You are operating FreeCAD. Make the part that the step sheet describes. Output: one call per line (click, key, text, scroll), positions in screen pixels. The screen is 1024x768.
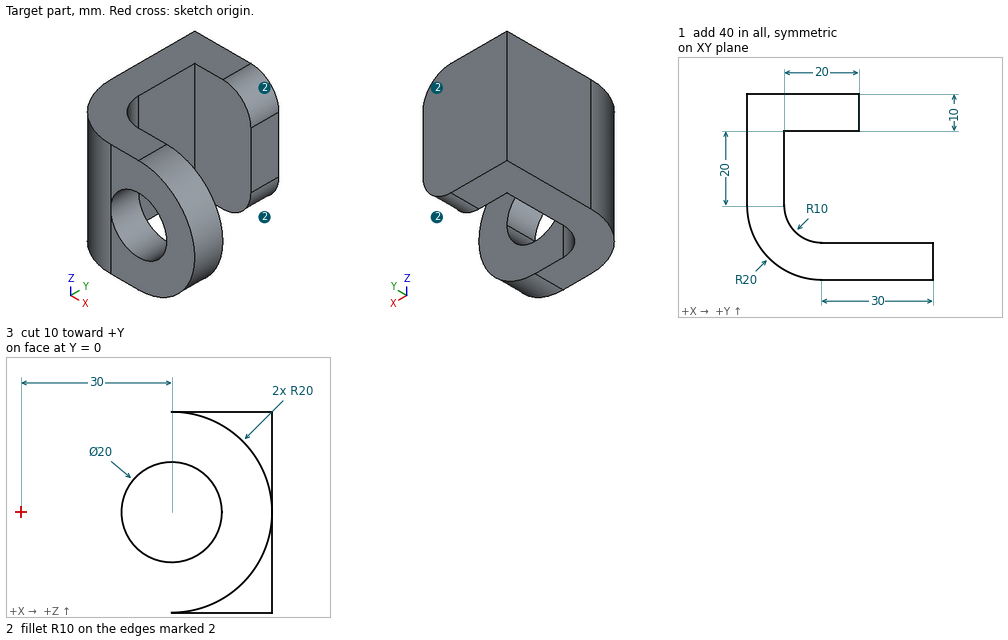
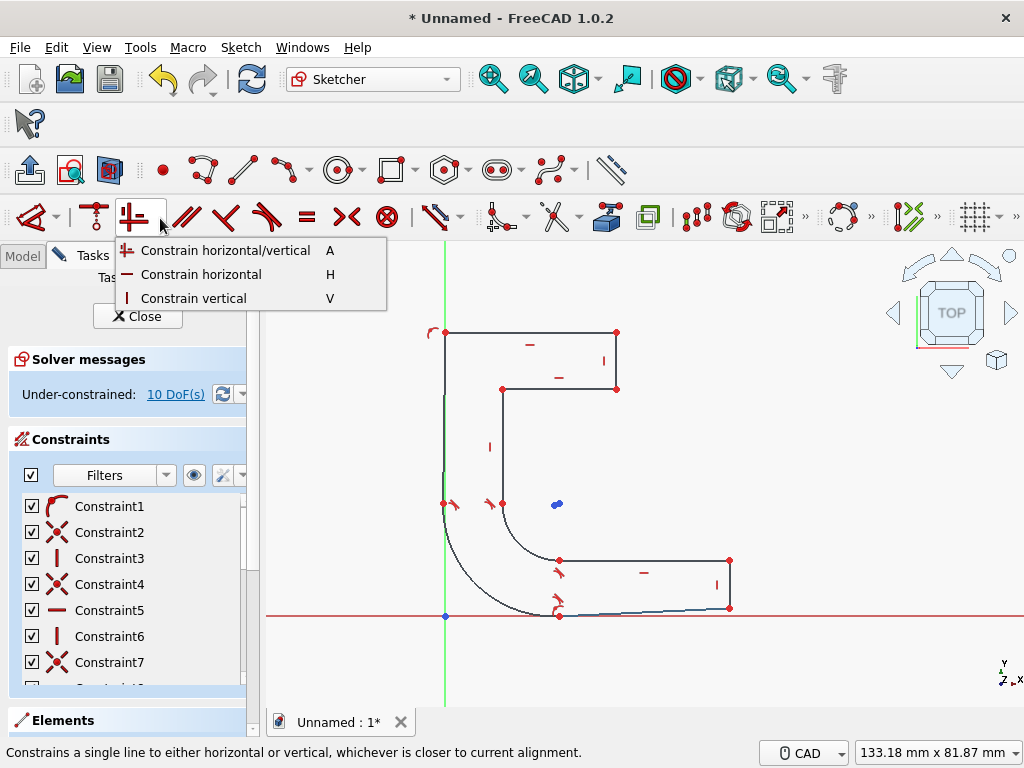
click(251, 274)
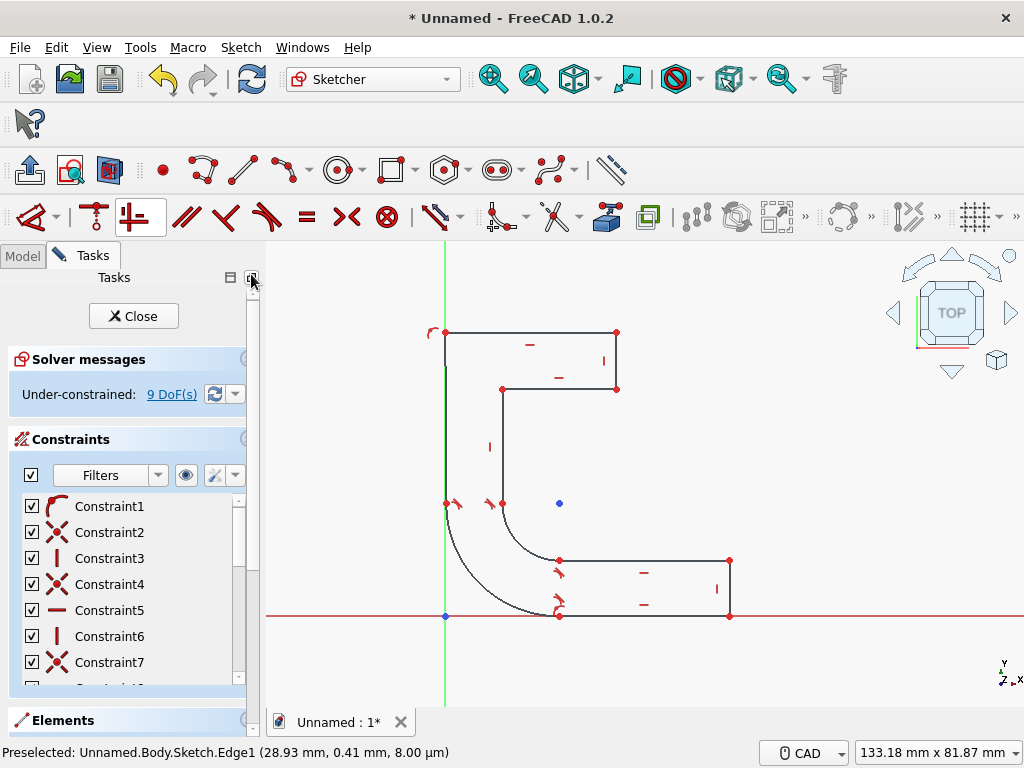
click(446, 384)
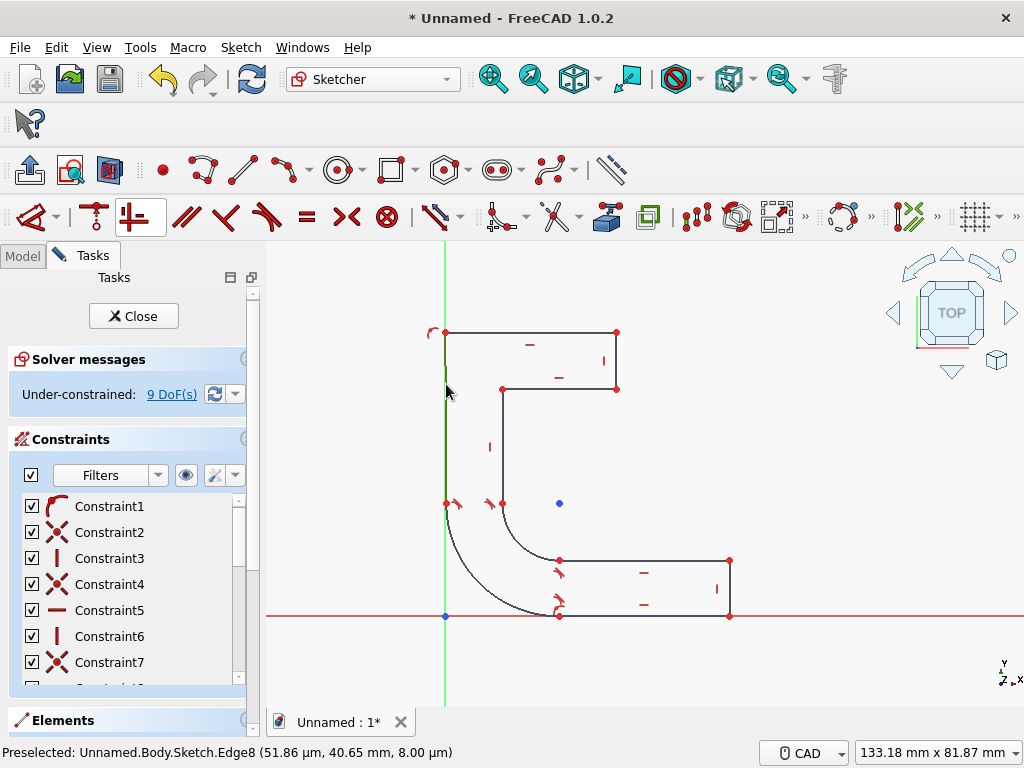
key(v)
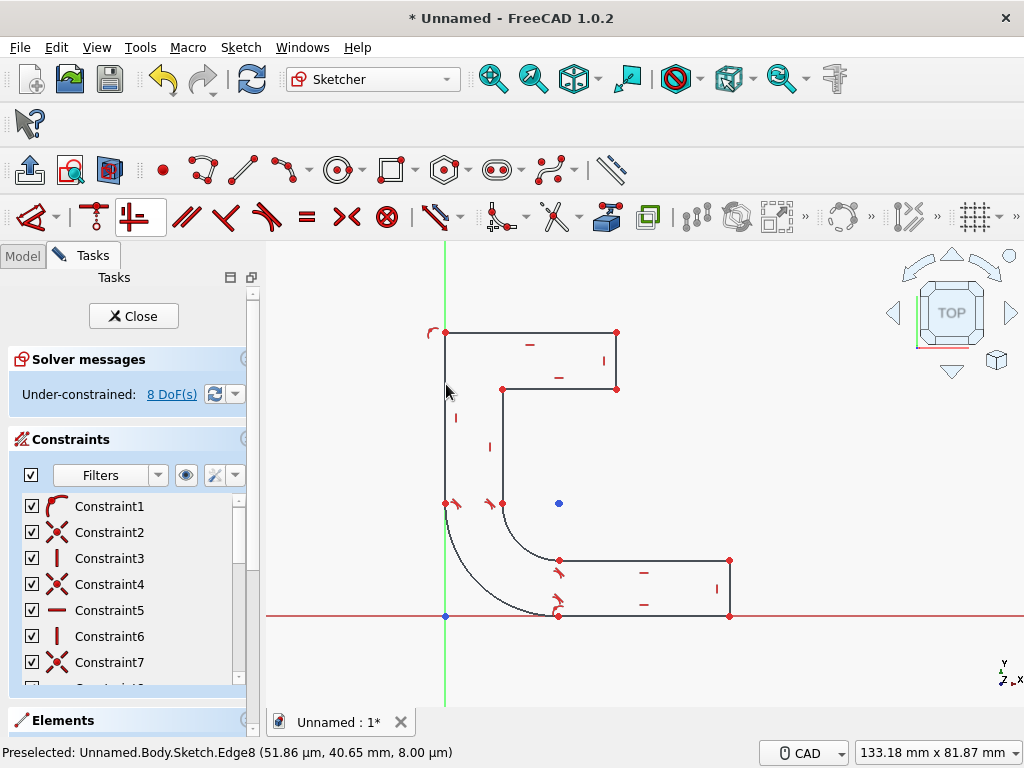
click(509, 530)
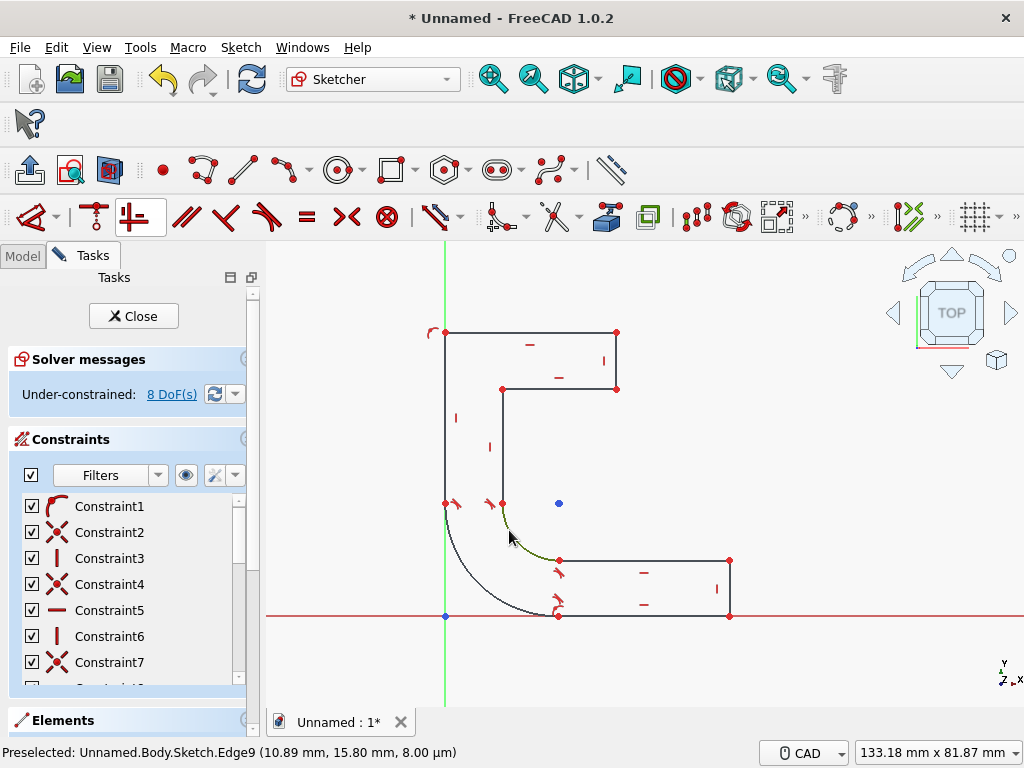
click(458, 555)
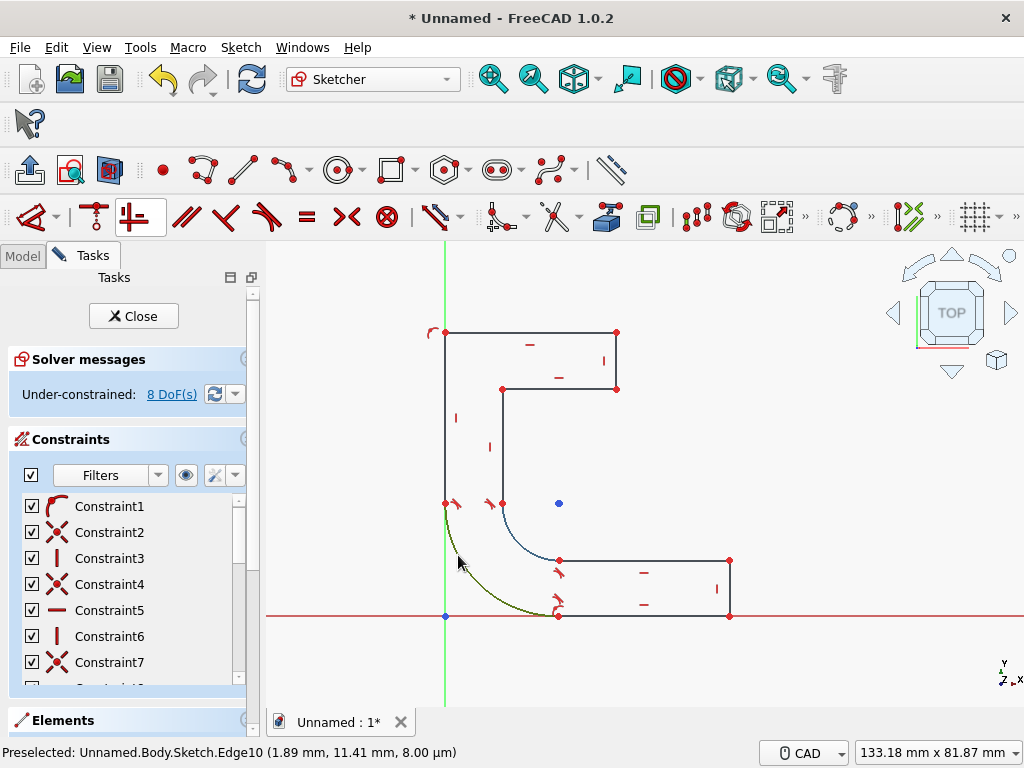
key(c)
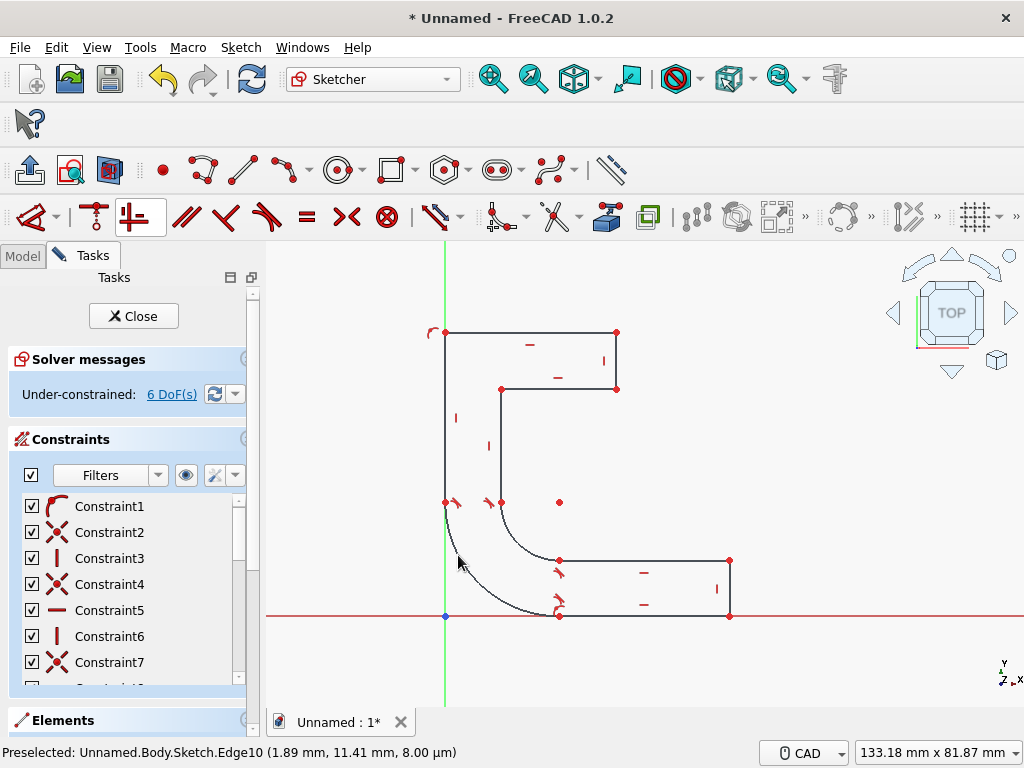
click(32, 218)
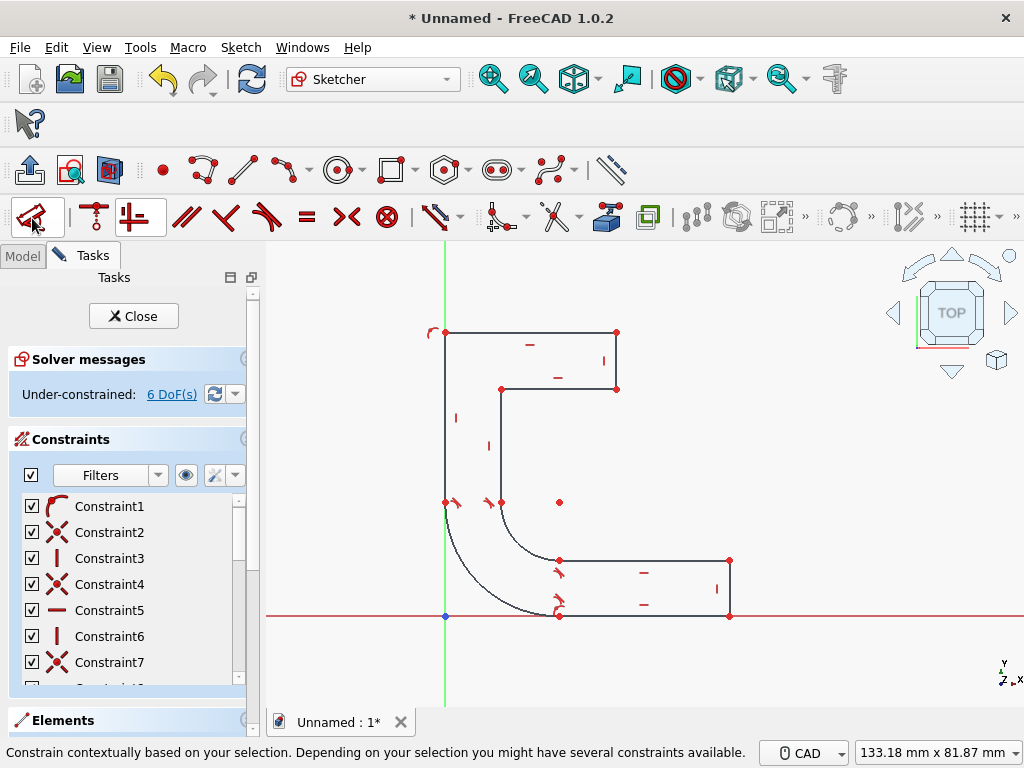
click(507, 529)
click(478, 544)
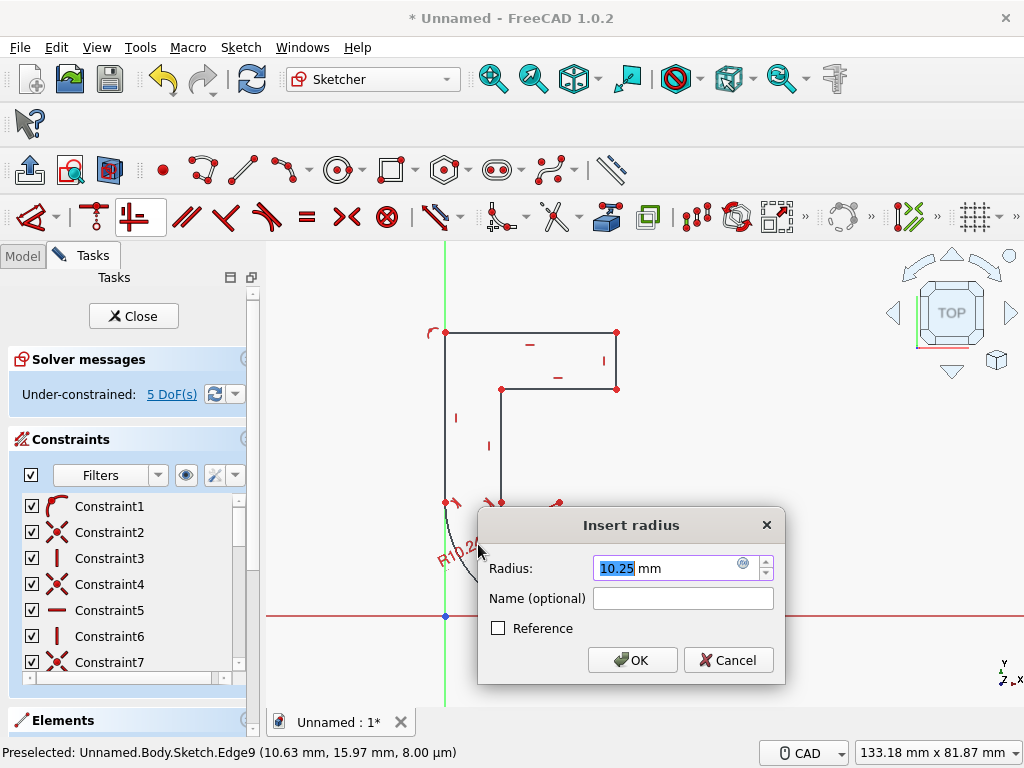
text(10)
key(Return)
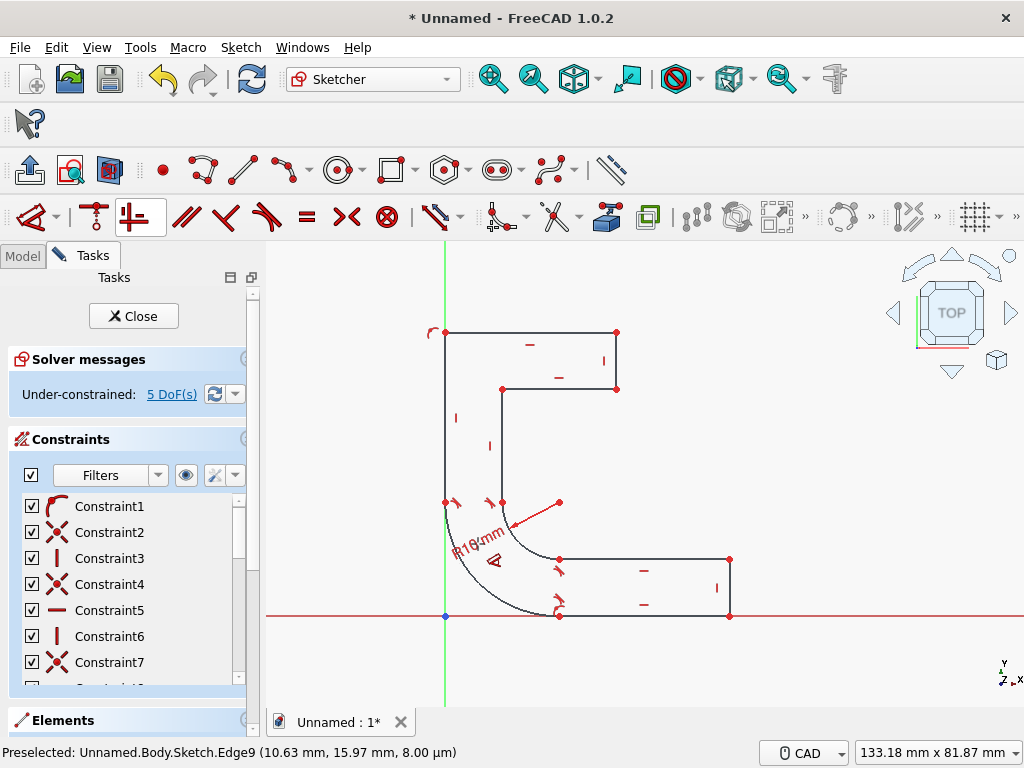
click(458, 554)
click(429, 569)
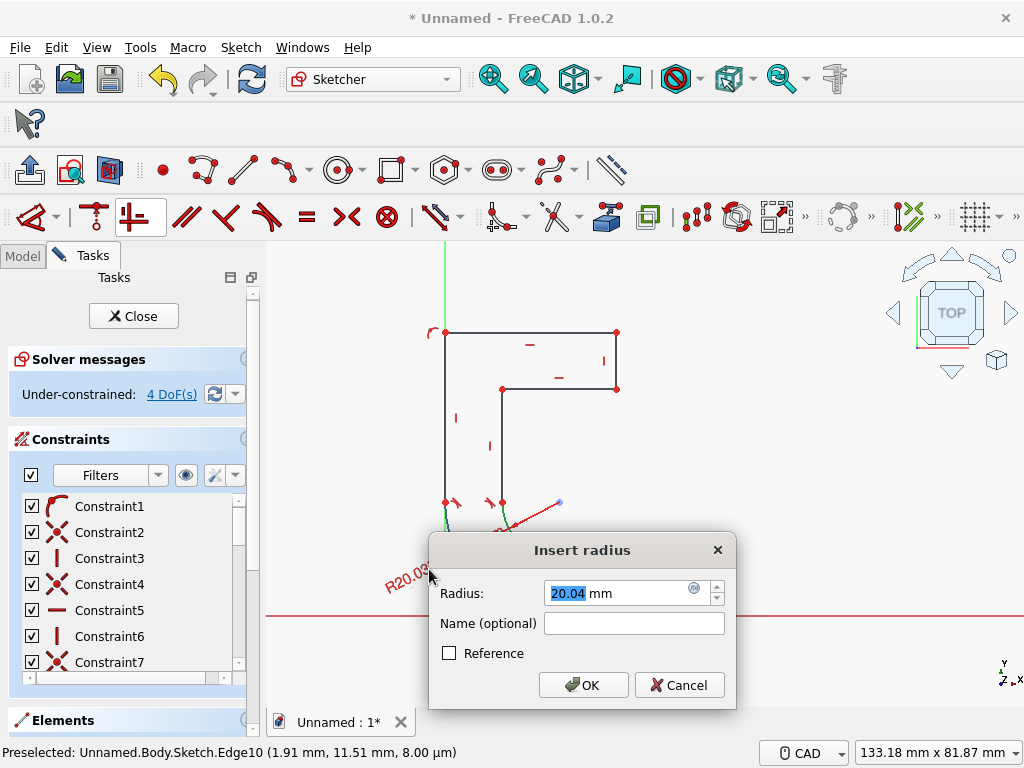
text(20)
key(Return)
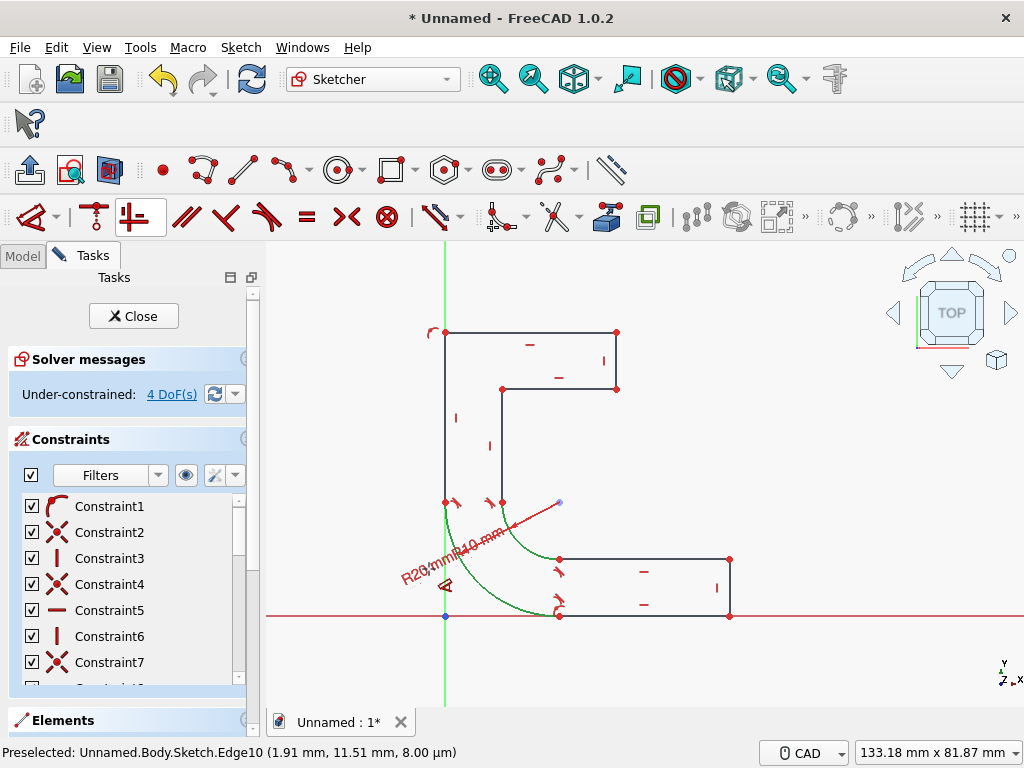
click(610, 616)
click(644, 650)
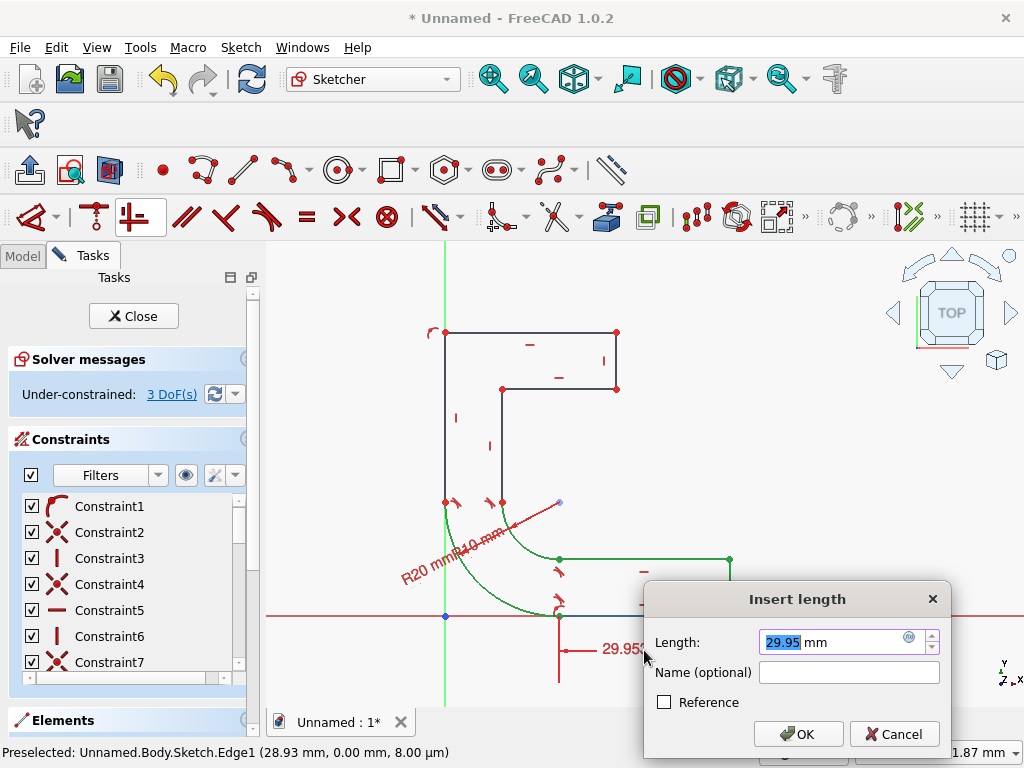
text(30)
key(Return)